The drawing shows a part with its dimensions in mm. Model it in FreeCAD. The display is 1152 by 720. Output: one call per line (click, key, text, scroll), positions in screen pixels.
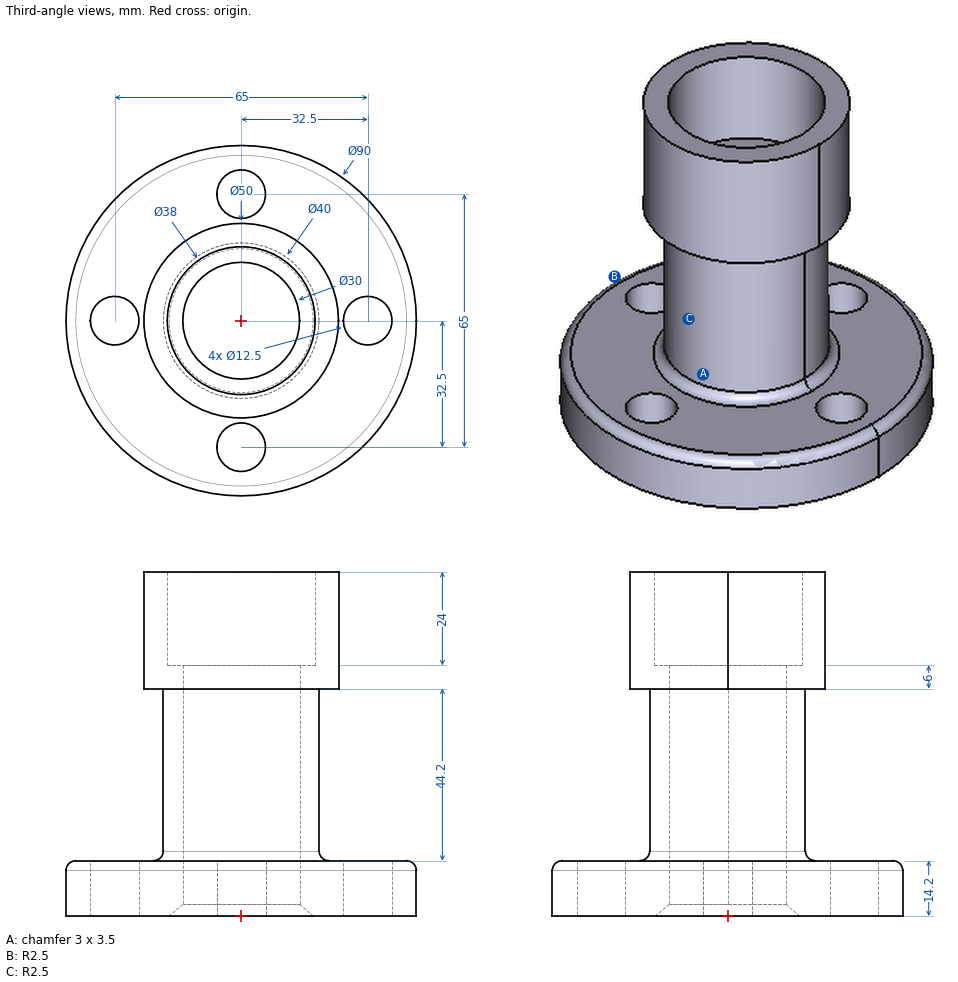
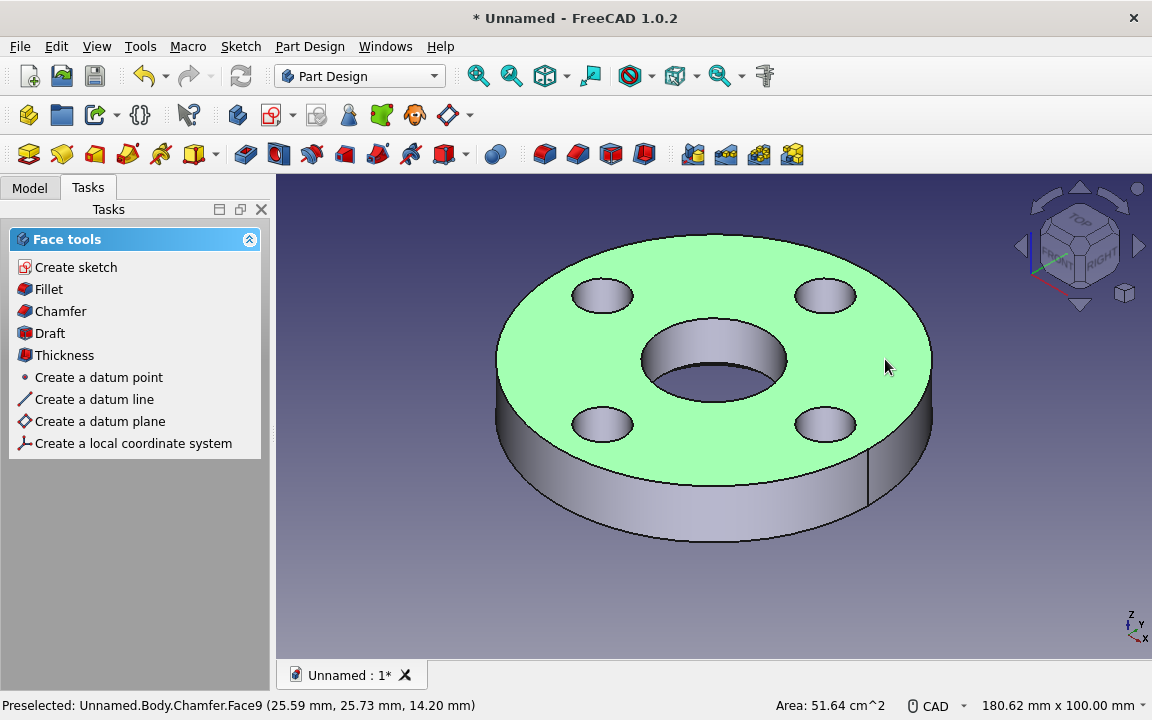
click(270, 116)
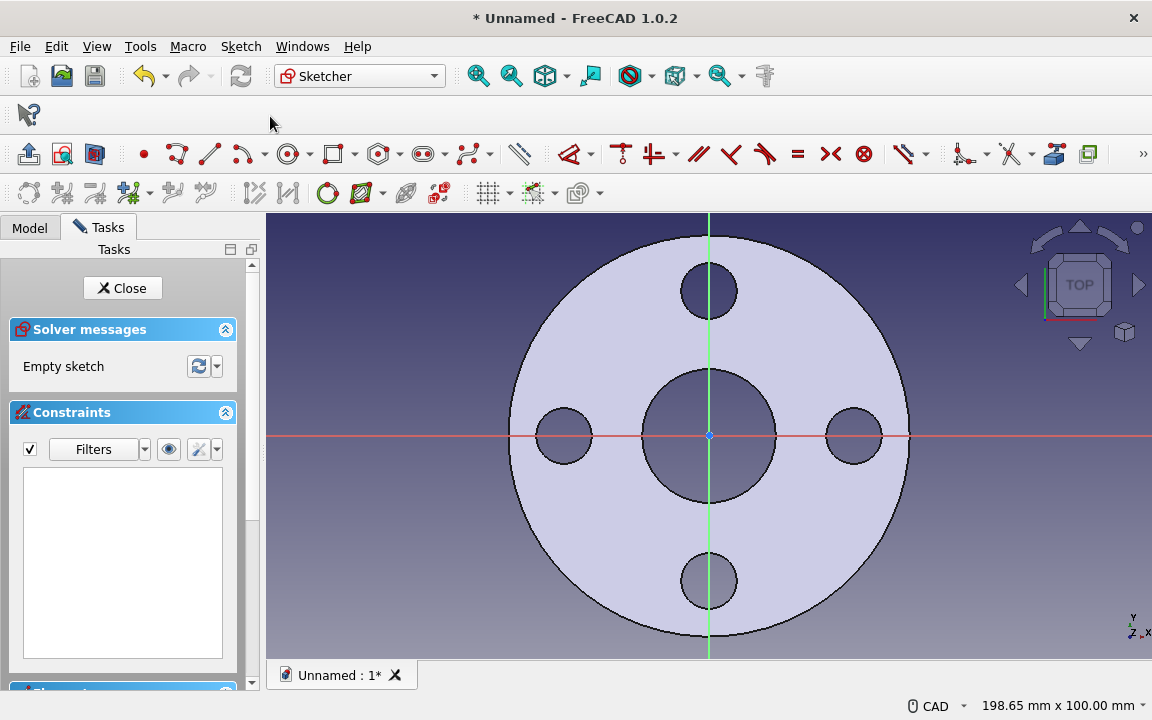
scroll(848, 436, up, 2)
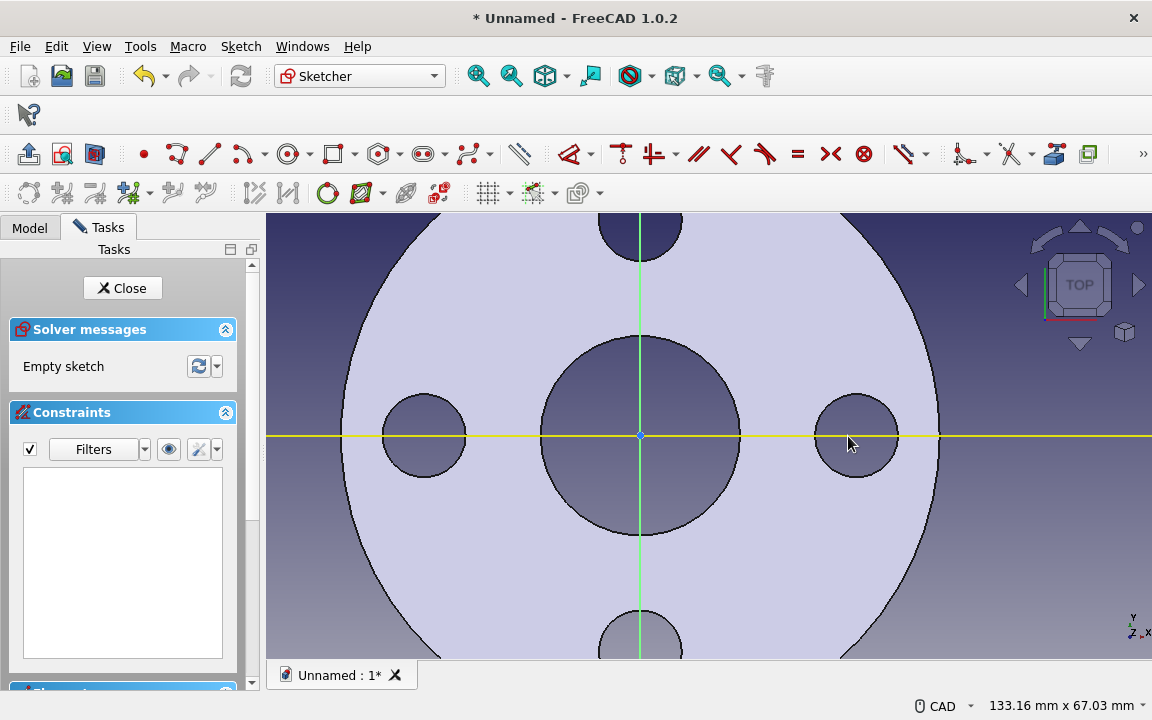
click(288, 154)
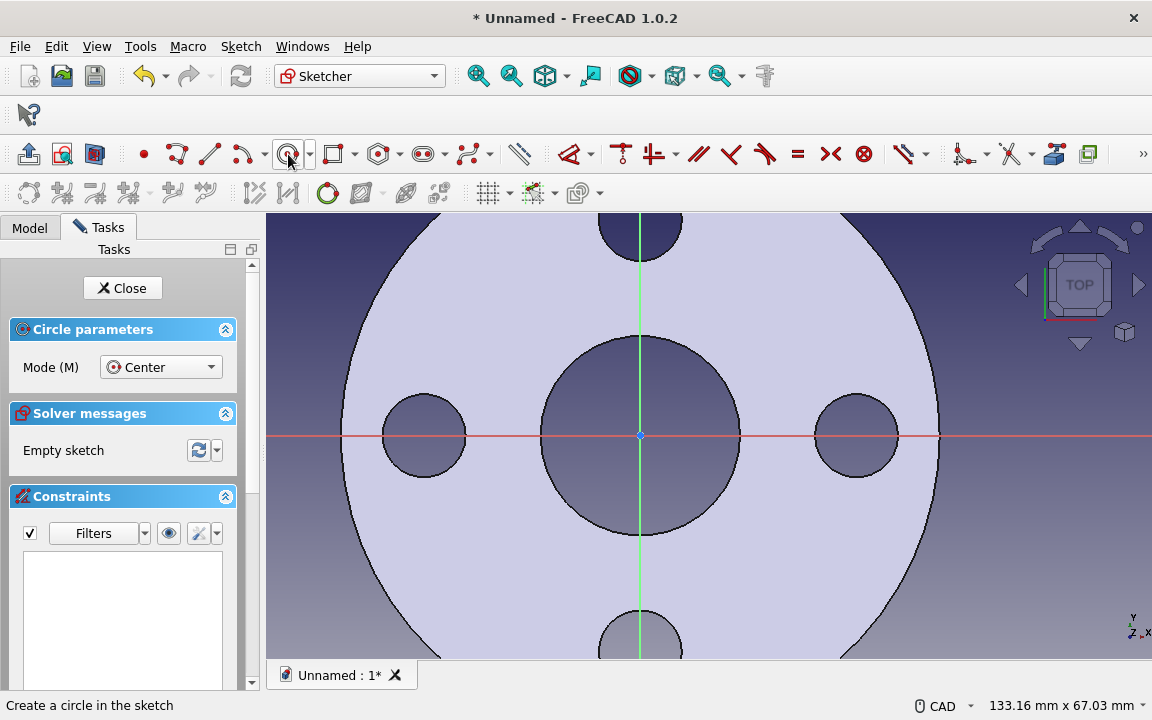
click(640, 436)
click(734, 342)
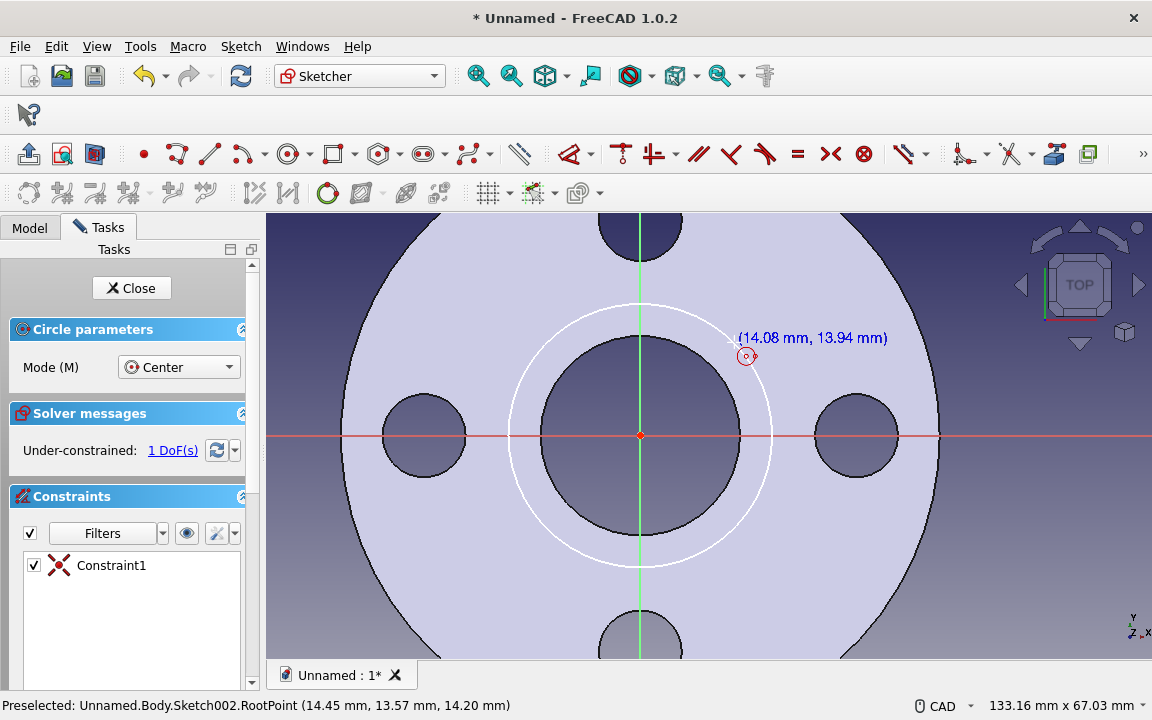
click(640, 436)
click(711, 365)
key(Escape)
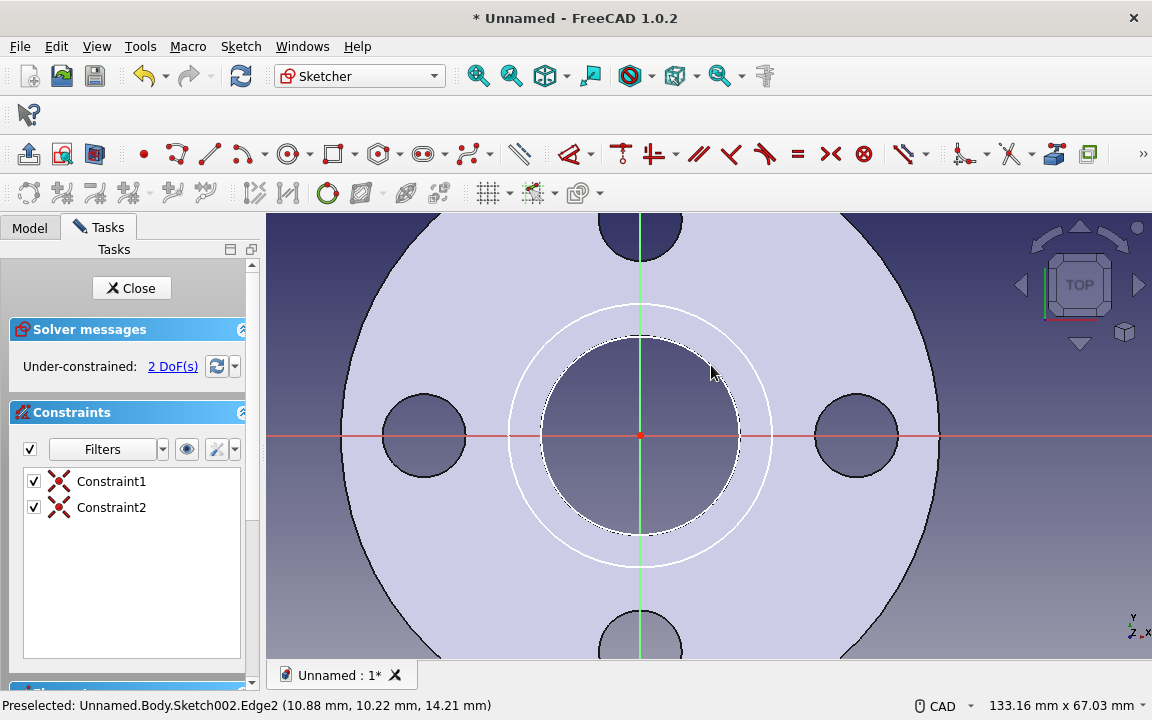
click(568, 154)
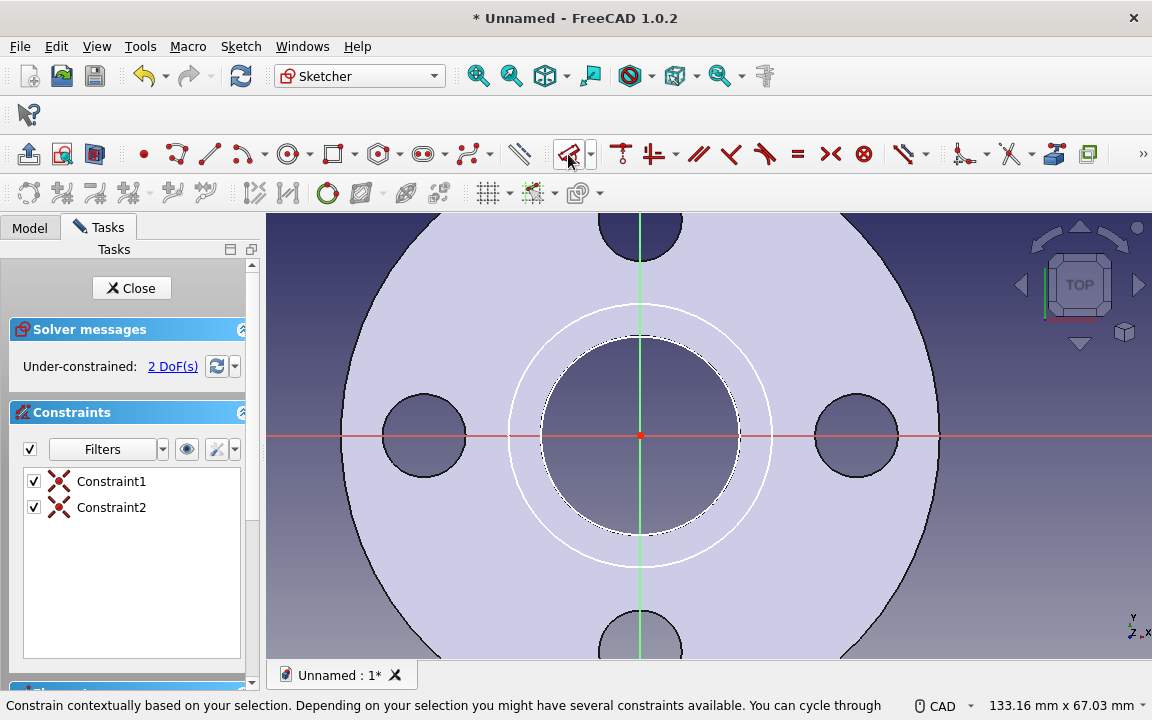
click(733, 342)
click(755, 319)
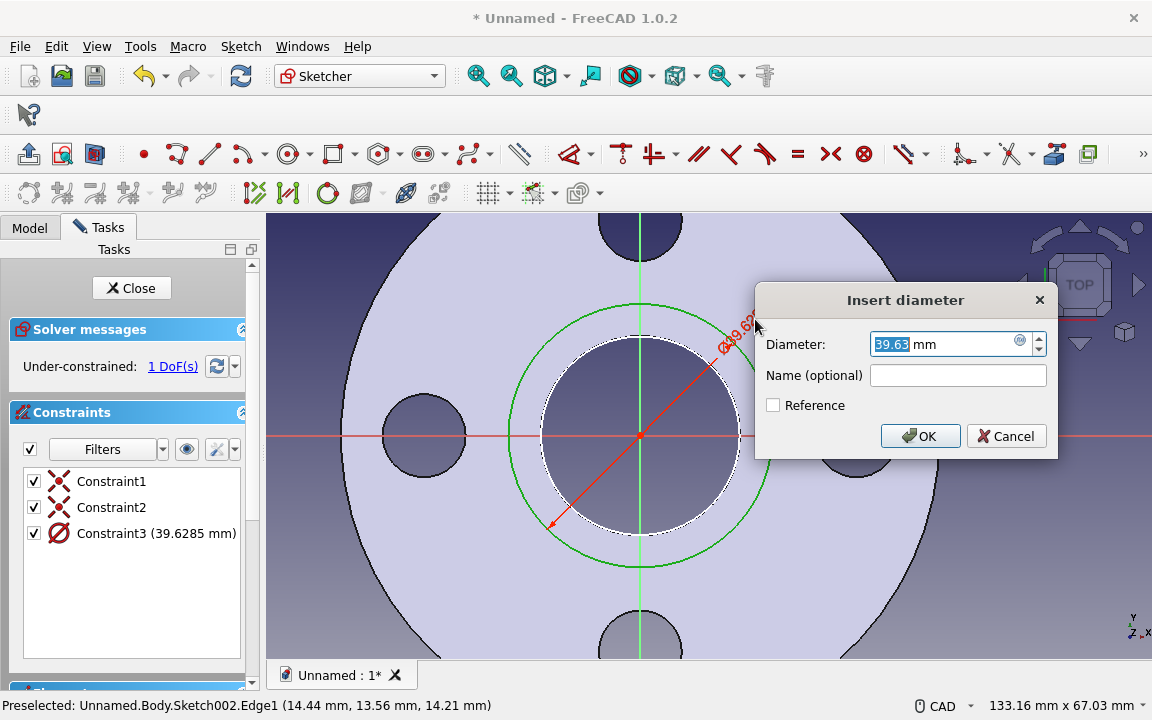
text(40)
key(Return)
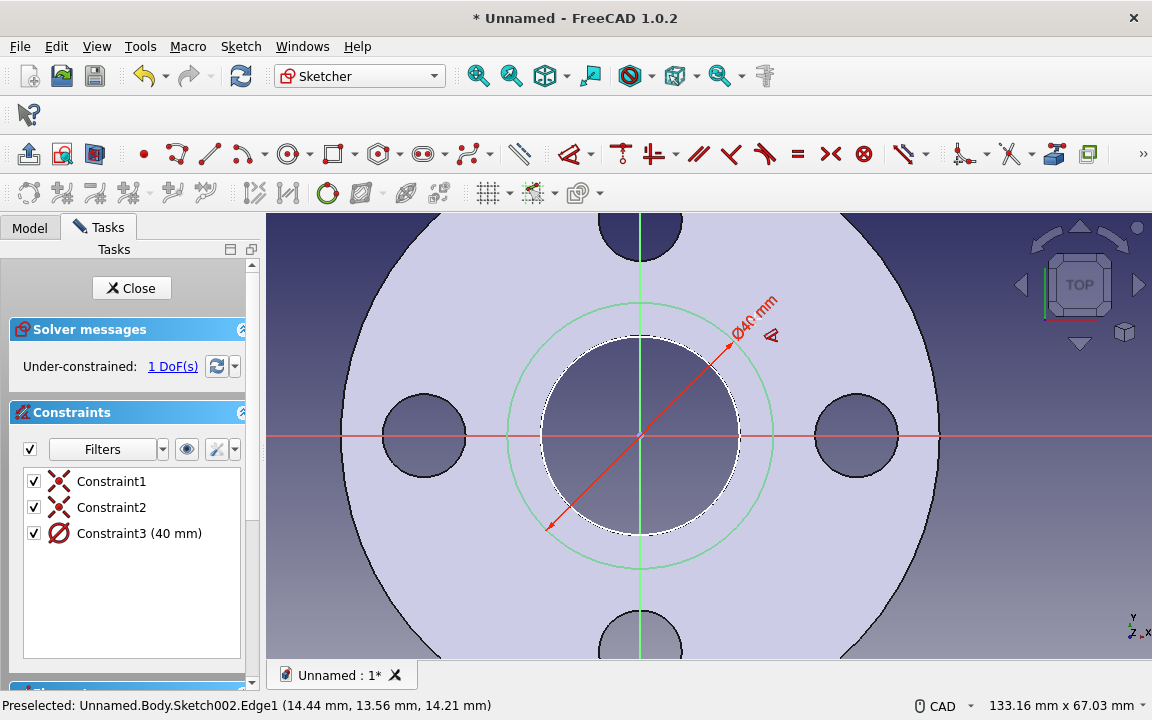
click(710, 365)
click(788, 391)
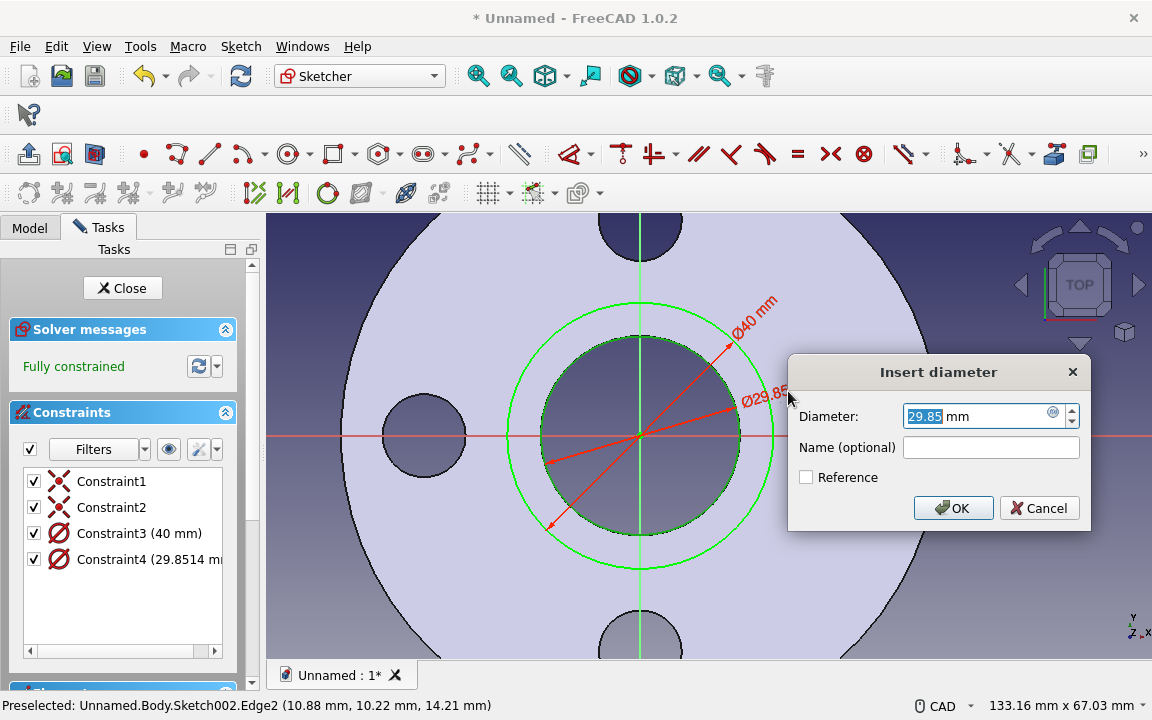
text(30)
key(Return)
key(Escape)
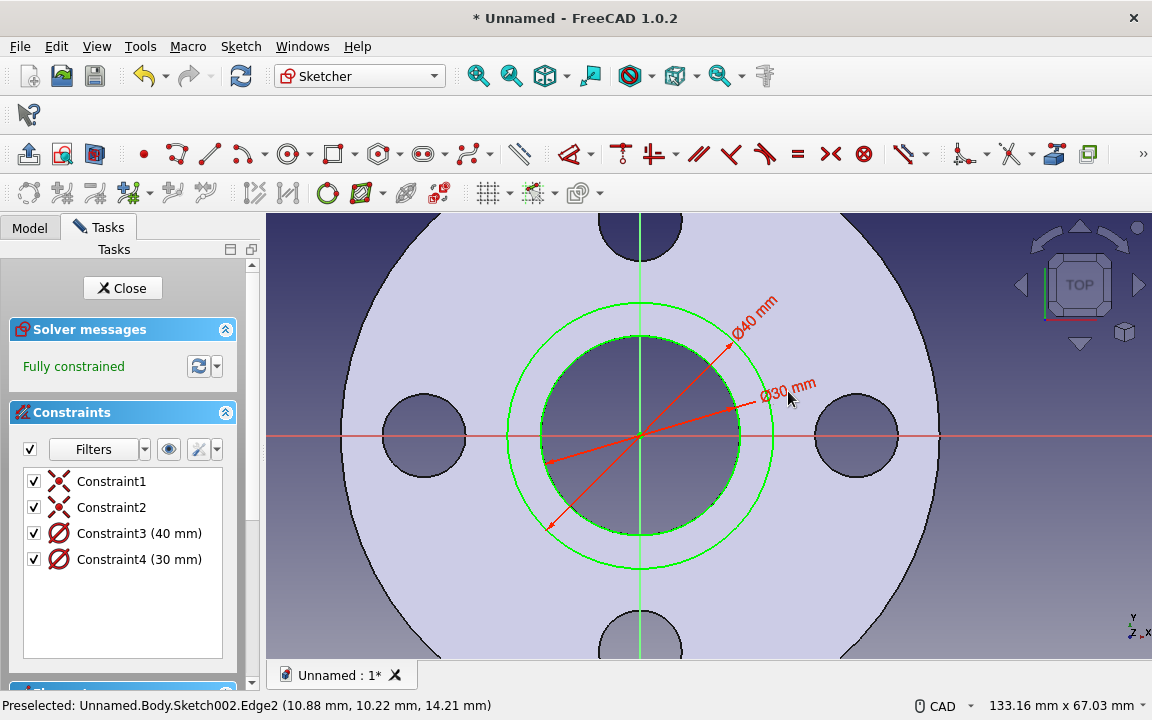
click(123, 288)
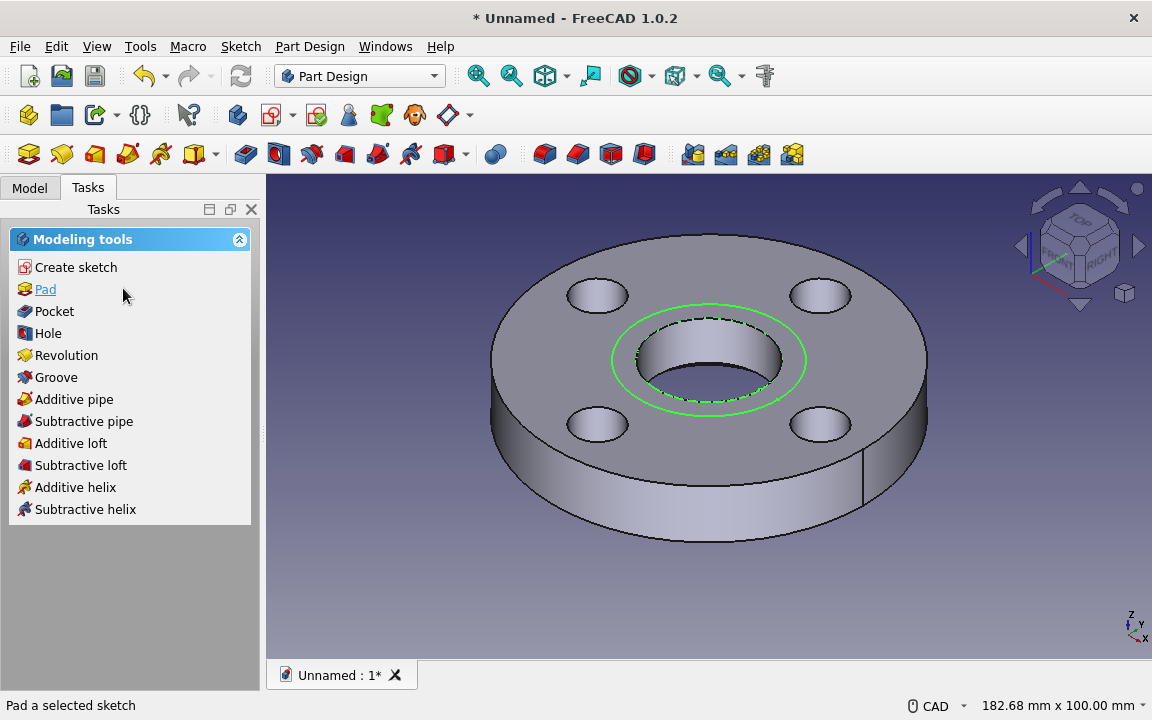
click(29, 154)